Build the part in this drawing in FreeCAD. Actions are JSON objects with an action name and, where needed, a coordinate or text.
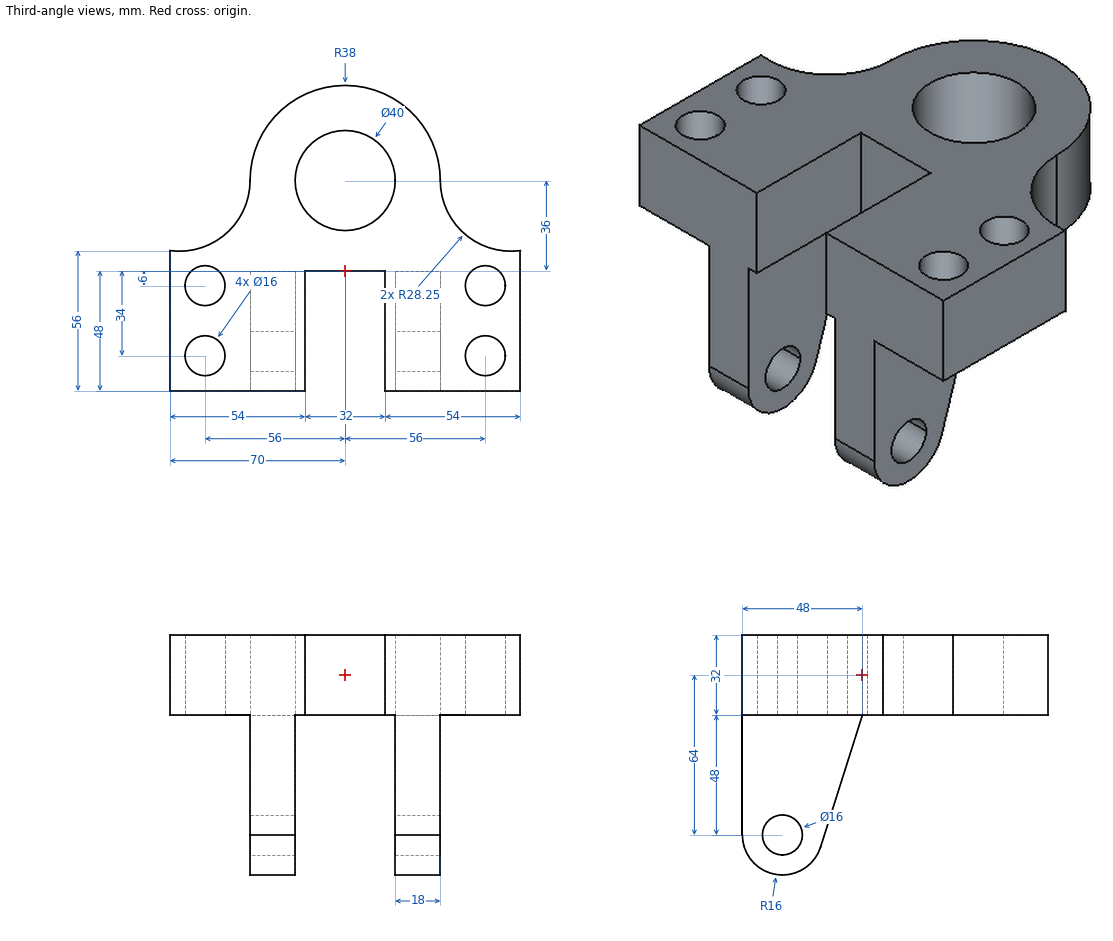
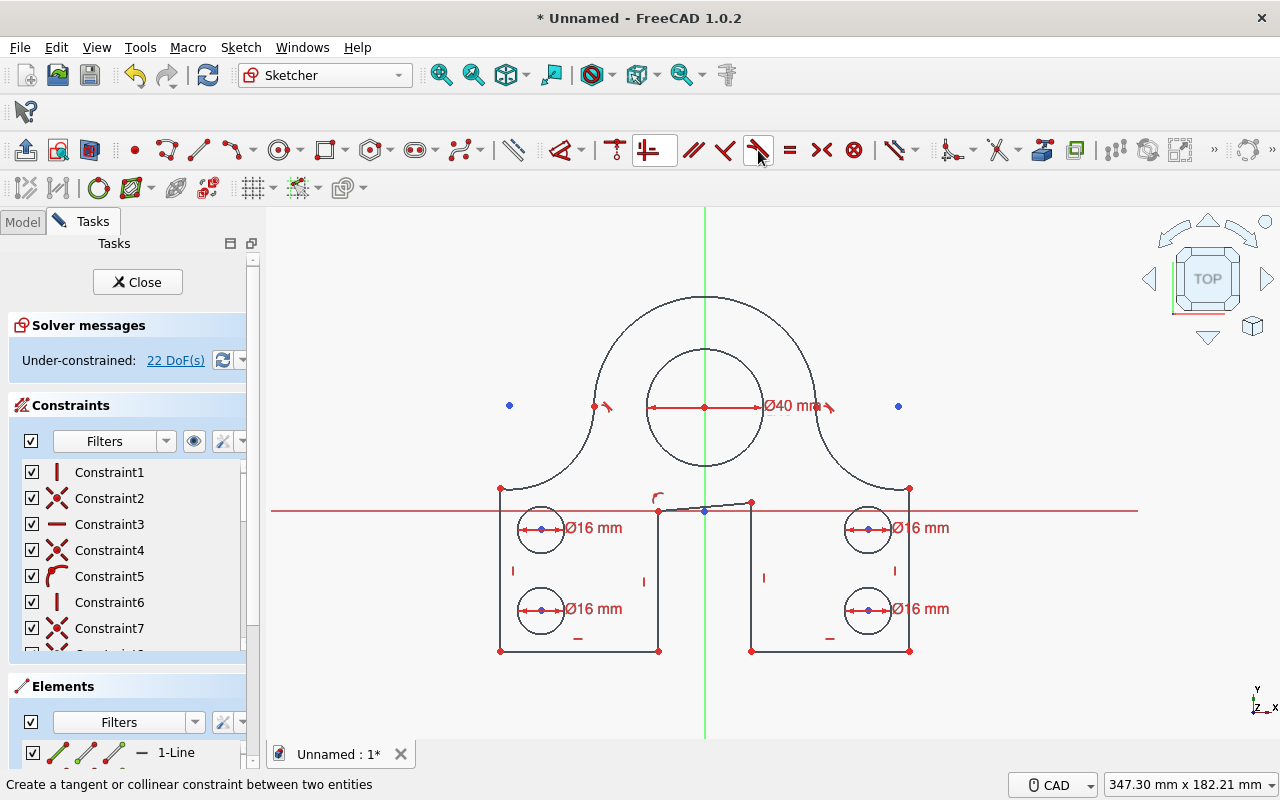
{"action": "left_click", "coordinate": [686, 509]}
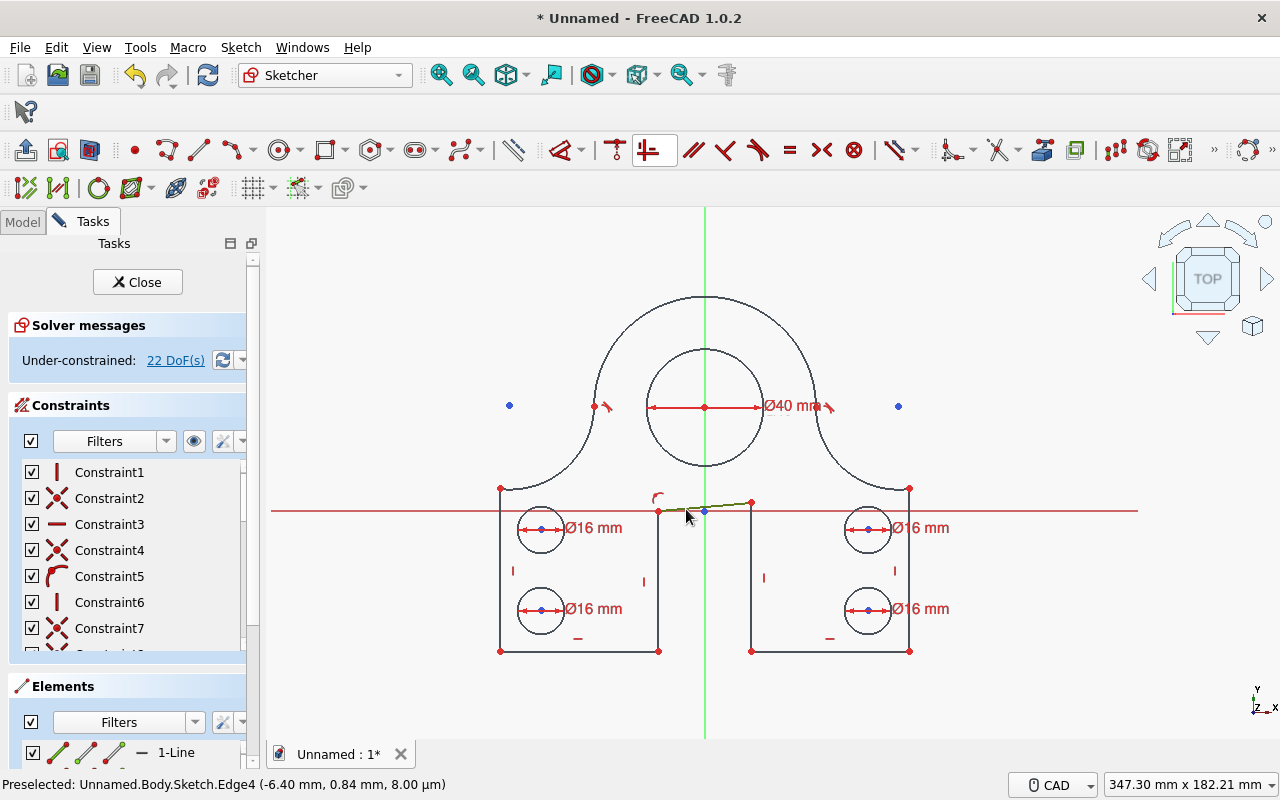
{"action": "left_click", "coordinate": [672, 150]}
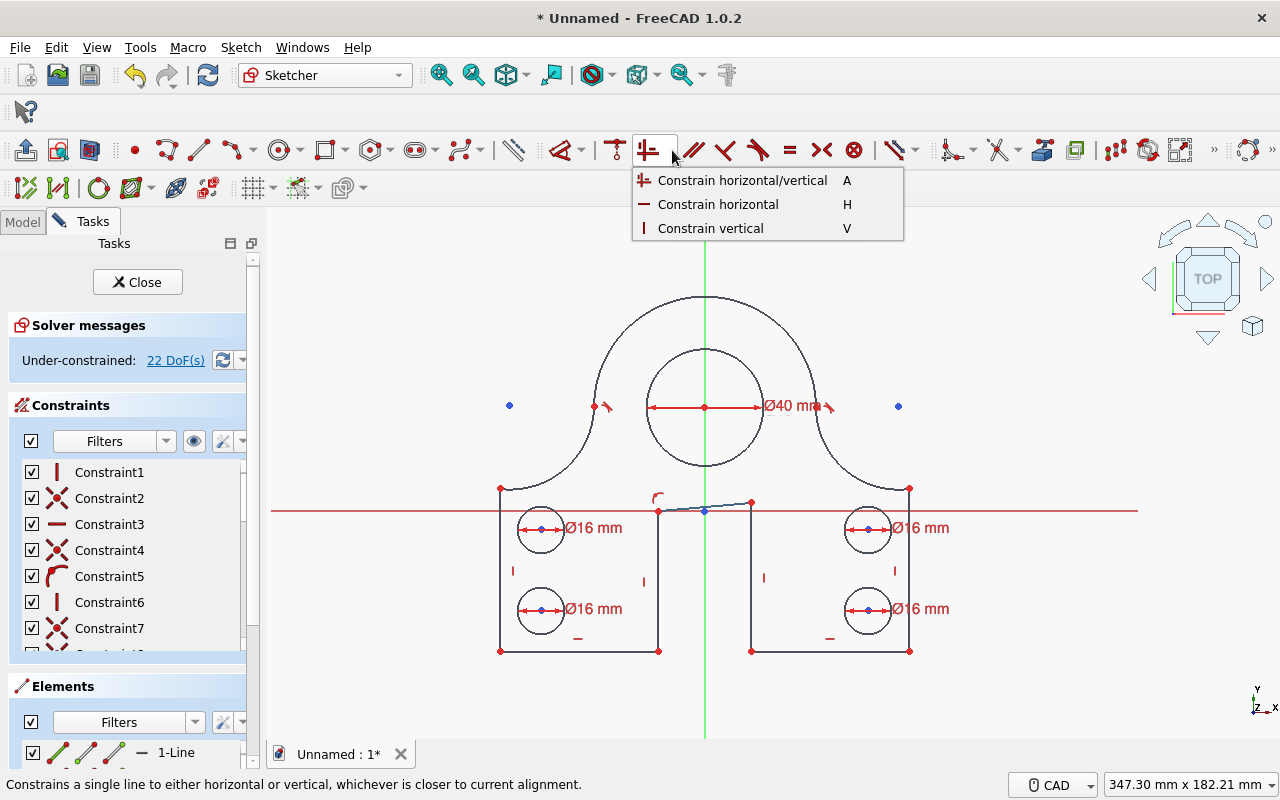
{"action": "left_click", "coordinate": [768, 204]}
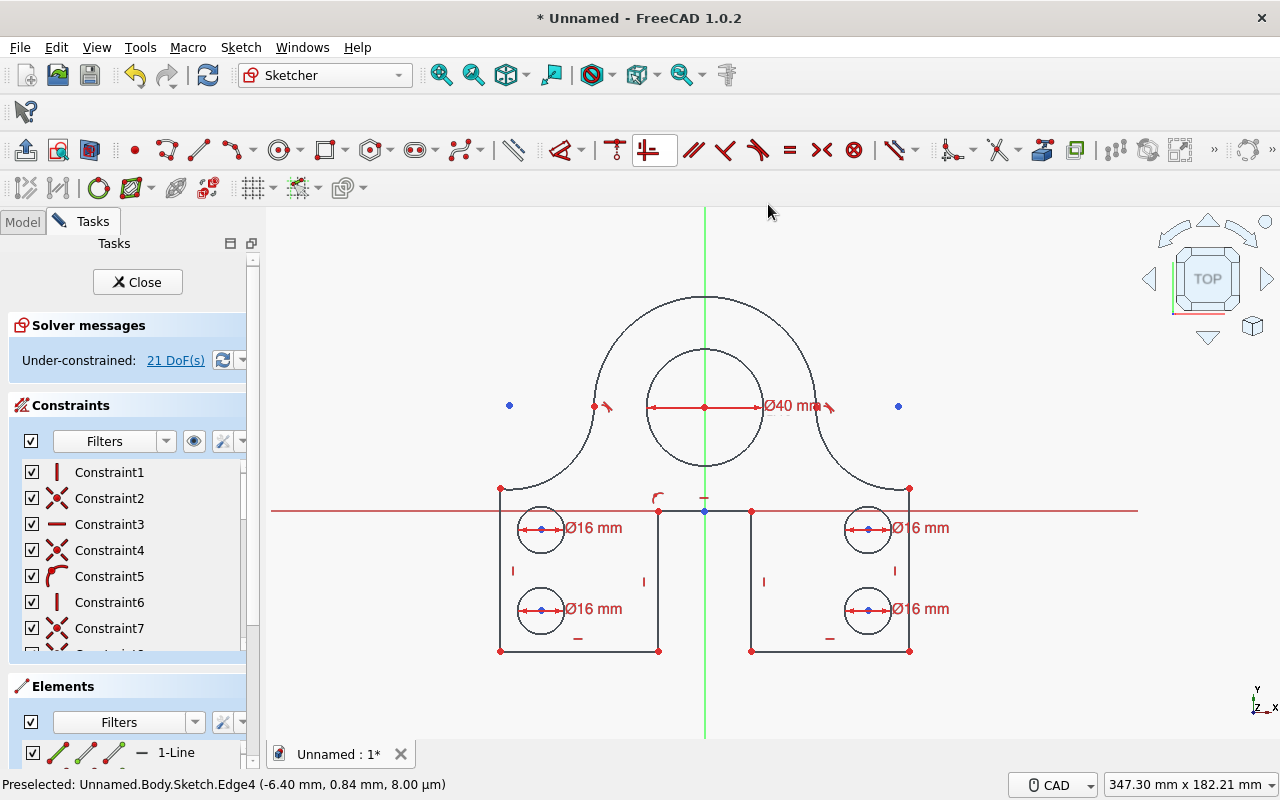
{"action": "left_click", "coordinate": [827, 447]}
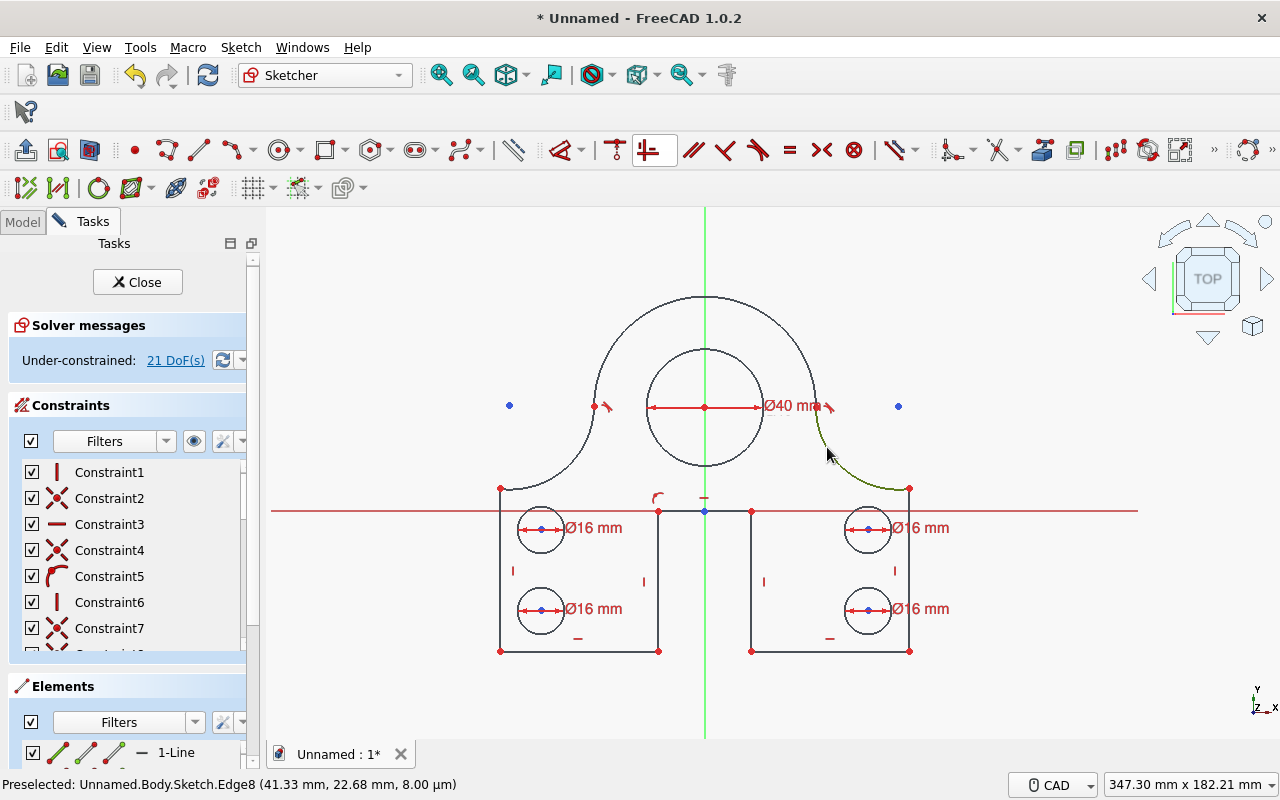
{"action": "left_click", "coordinate": [542, 483]}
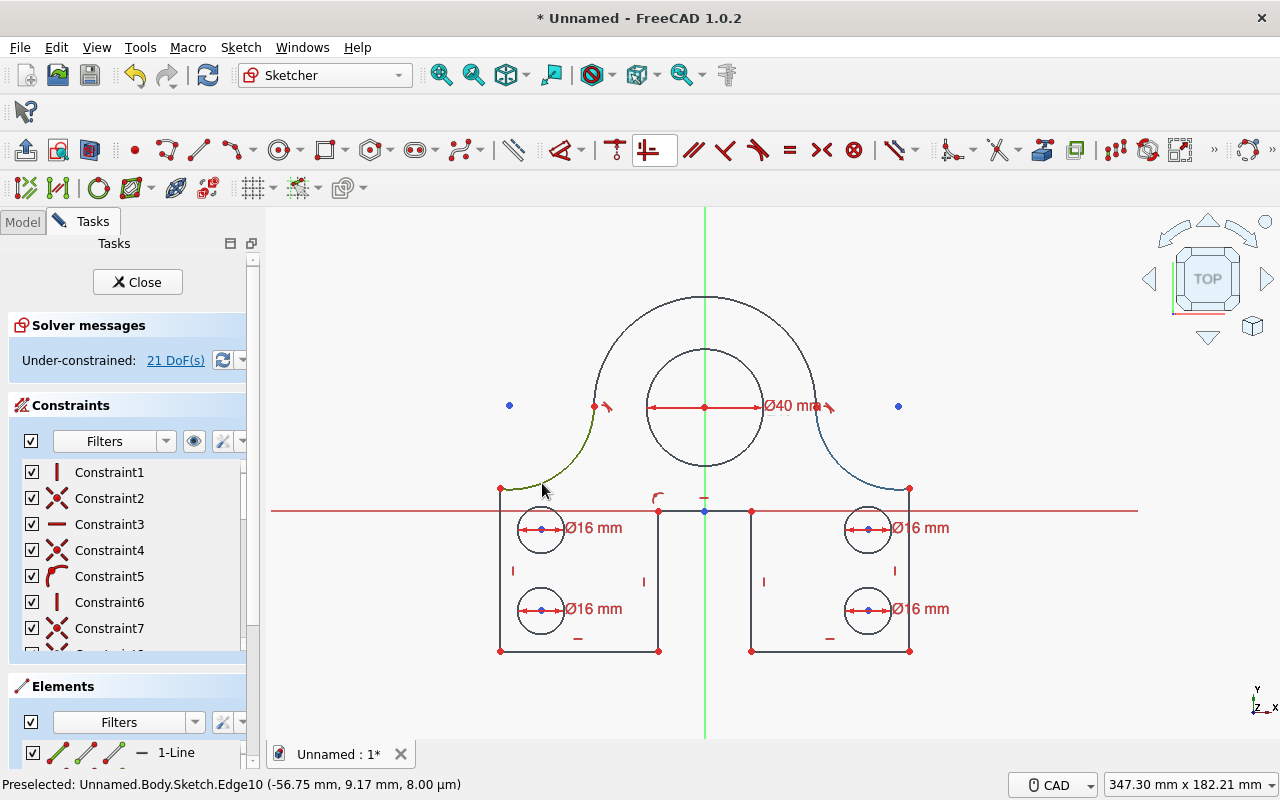
{"action": "left_click", "coordinate": [790, 150]}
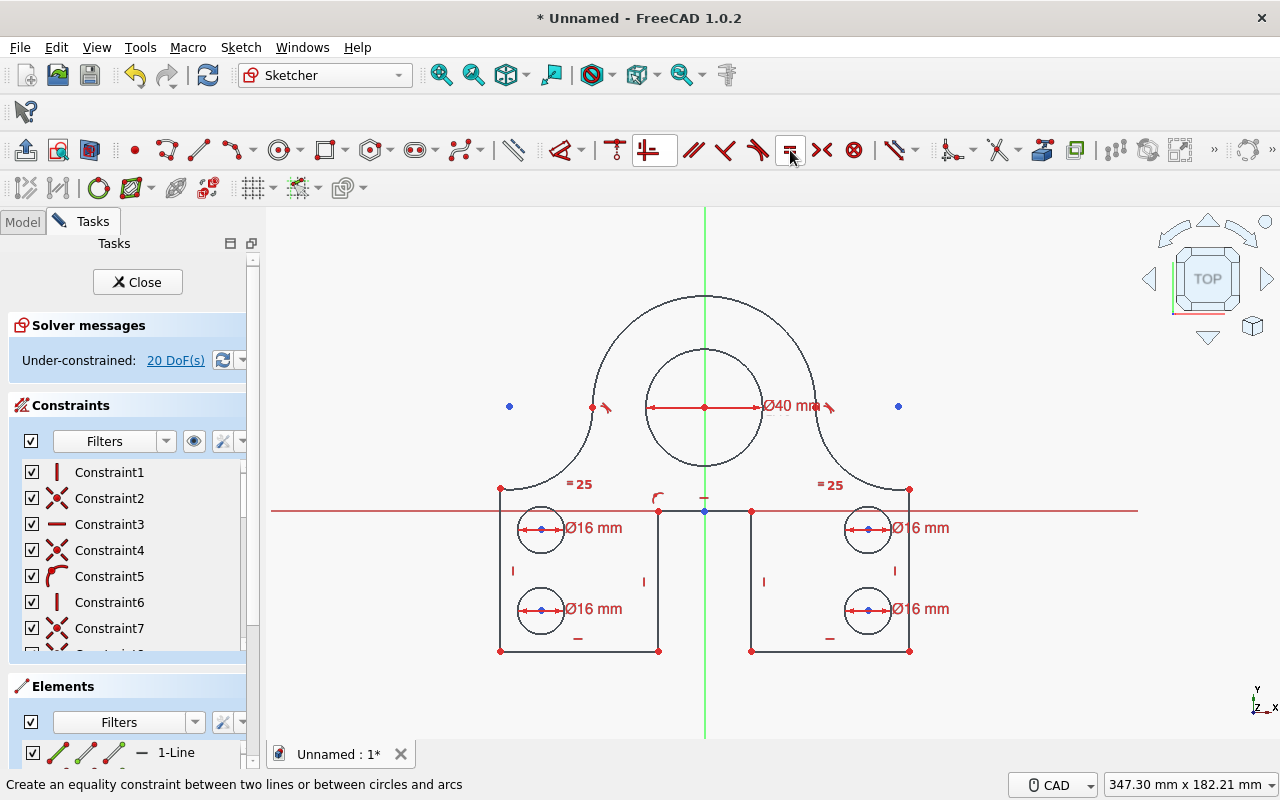
{"action": "left_click", "coordinate": [704, 408]}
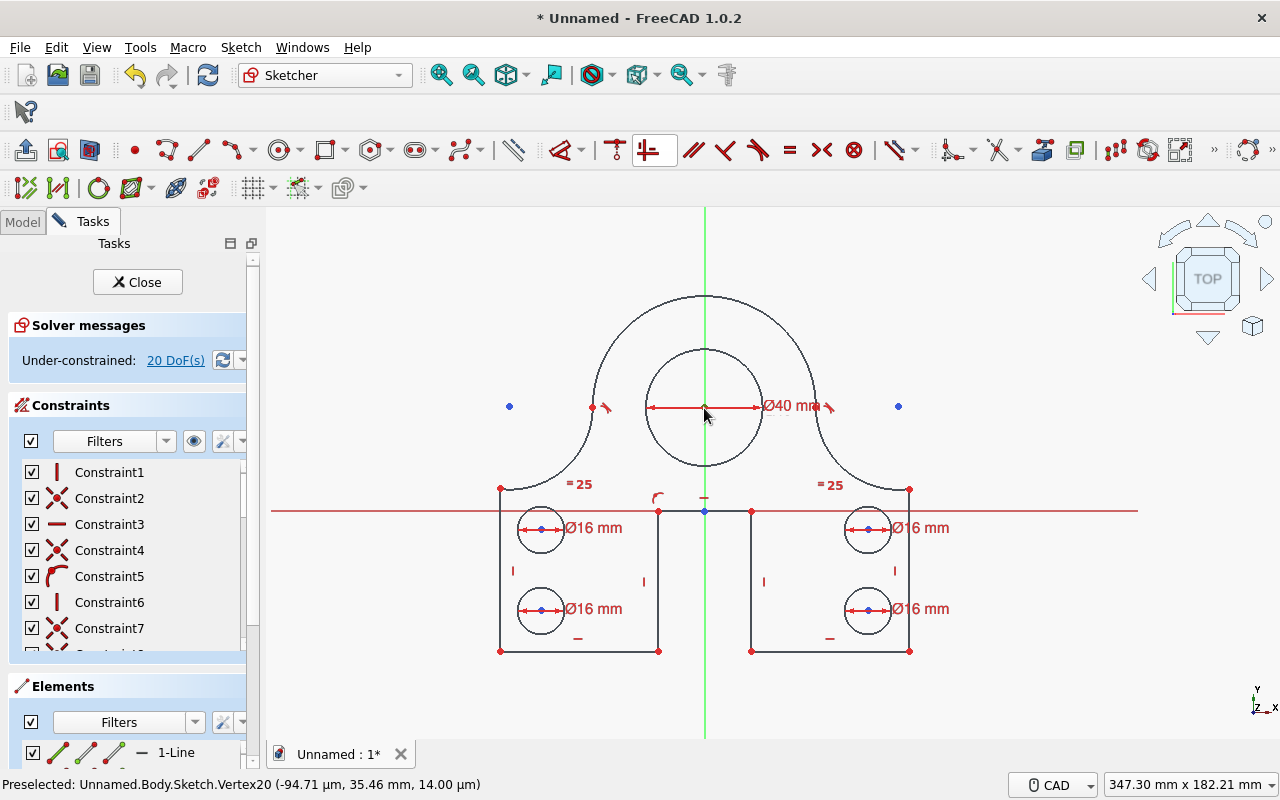
{"action": "left_click", "coordinate": [705, 677]}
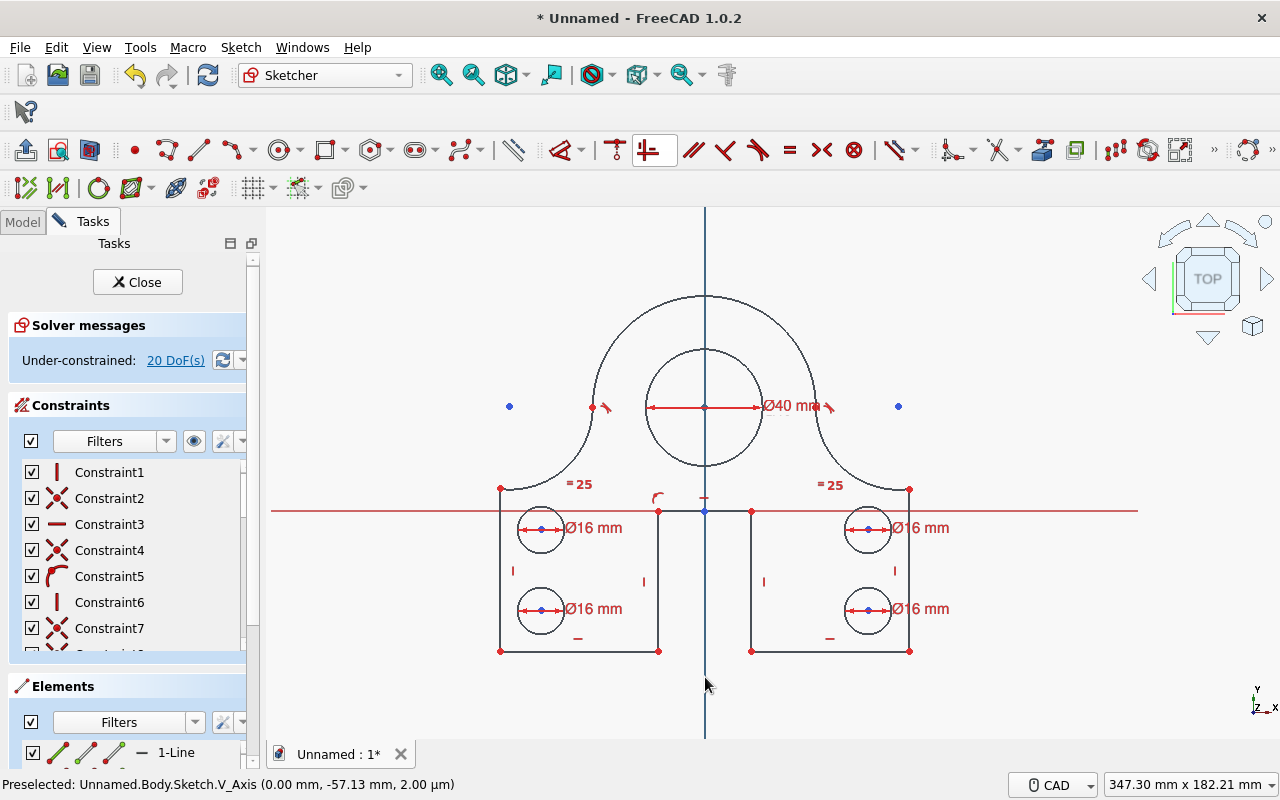
{"action": "left_click", "coordinate": [616, 150]}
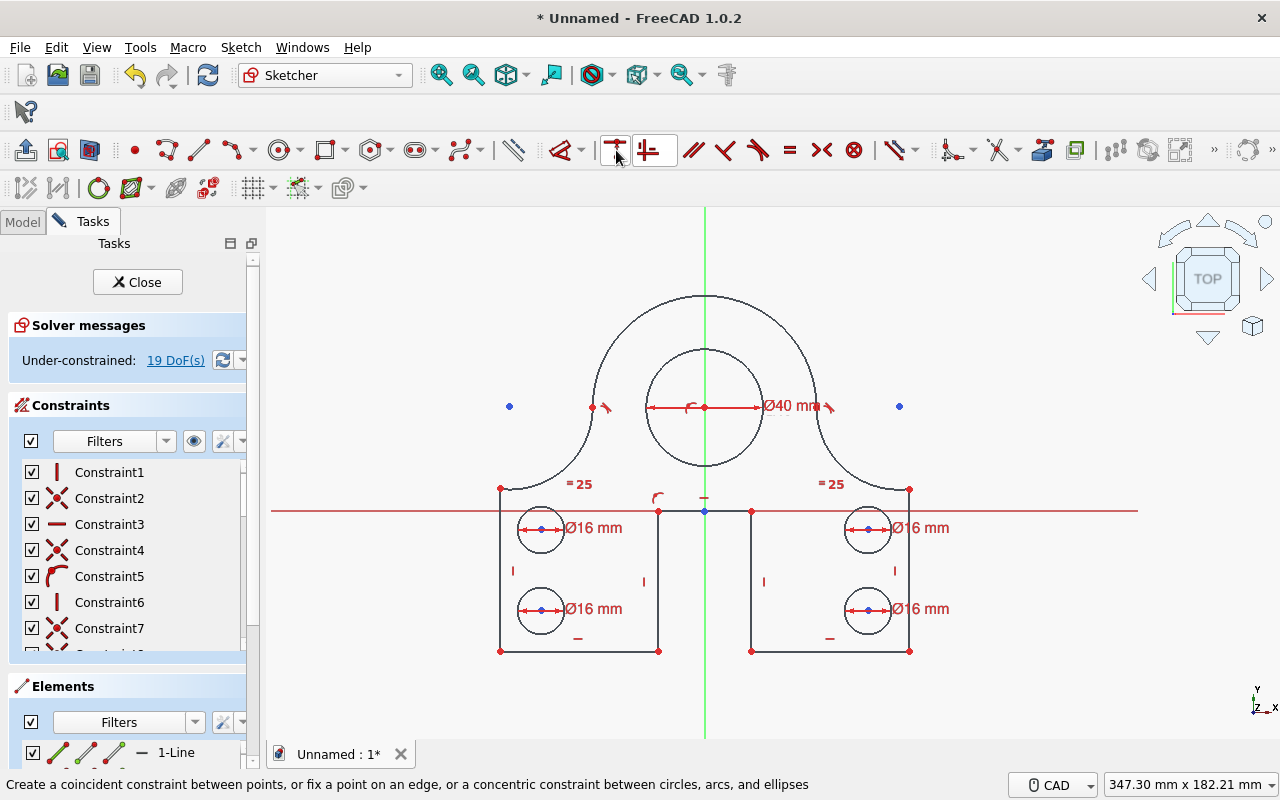
{"action": "left_click", "coordinate": [541, 611]}